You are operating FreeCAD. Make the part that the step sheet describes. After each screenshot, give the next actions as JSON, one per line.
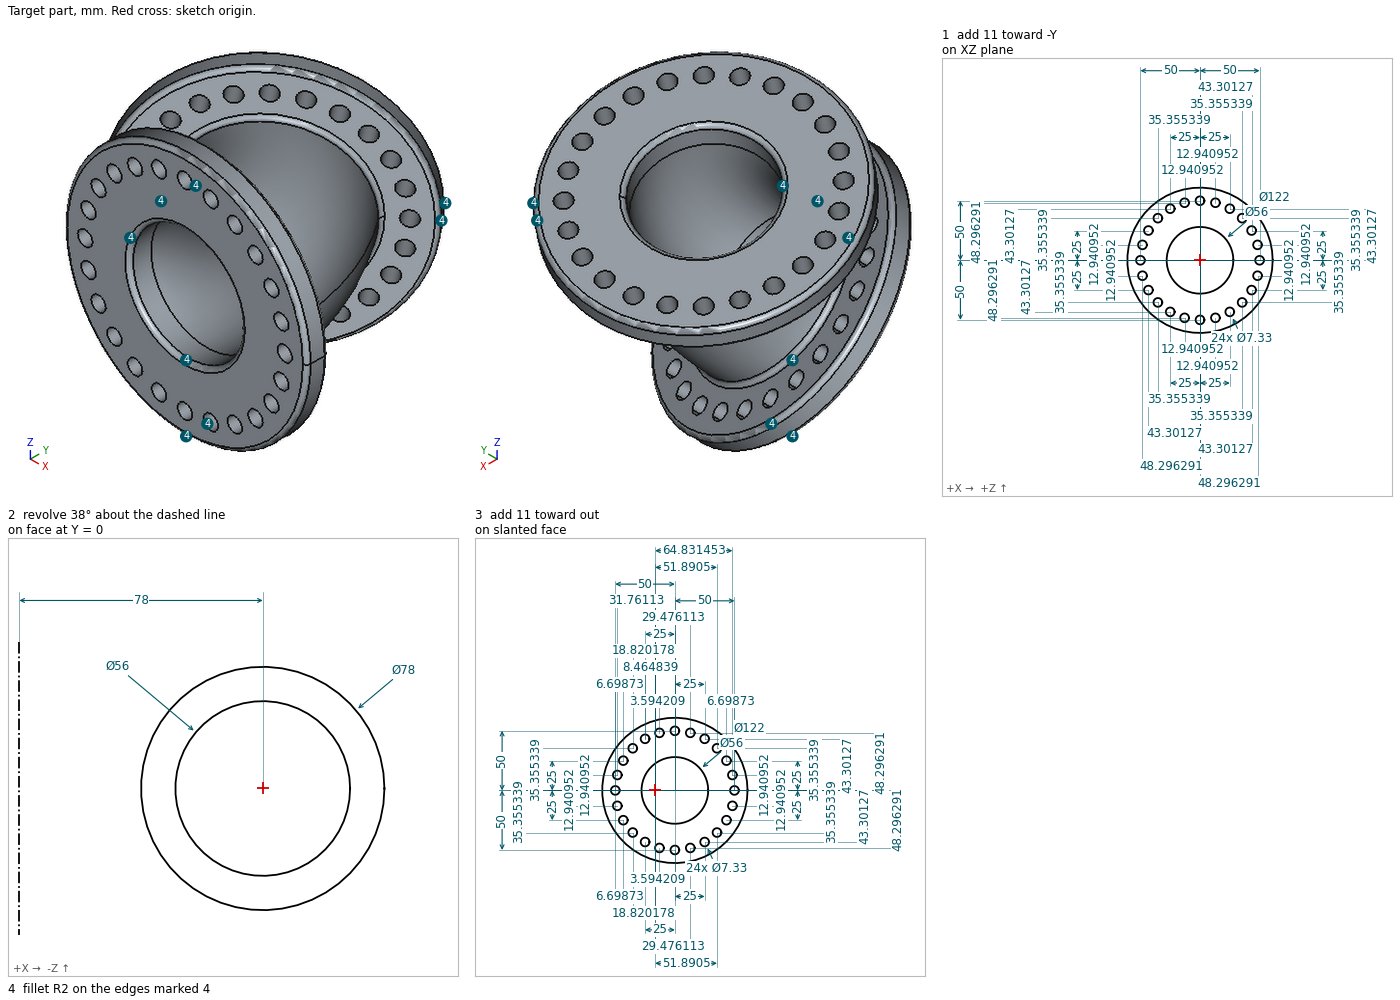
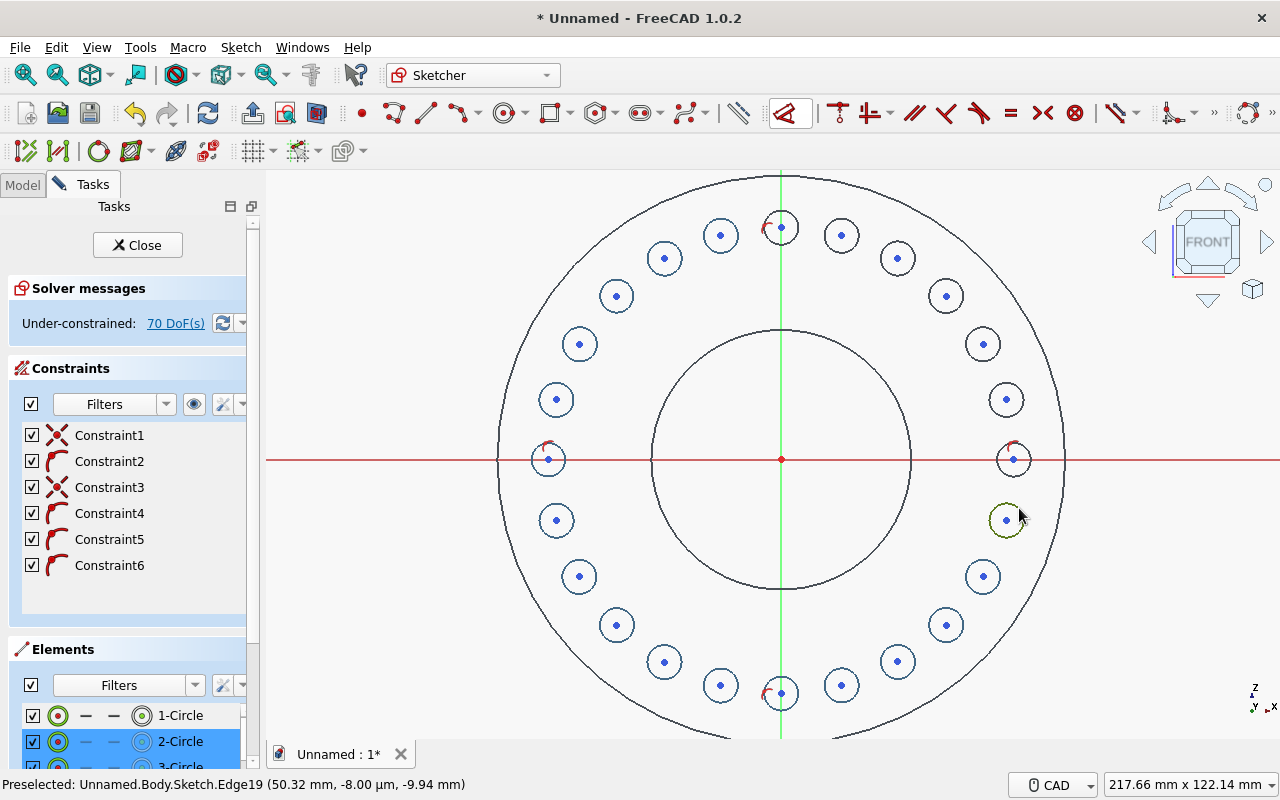
{"action": "left_click", "coordinate": [1026, 448]}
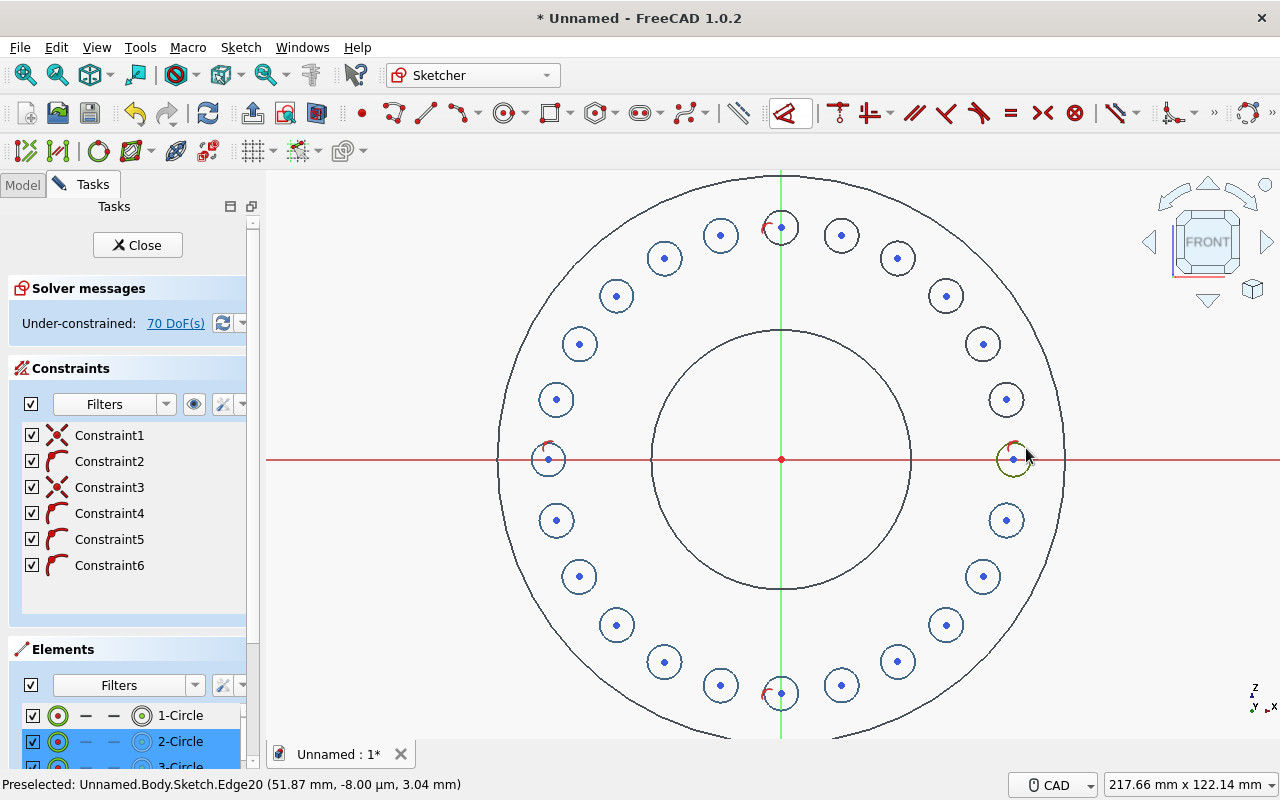
{"action": "left_click", "coordinate": [793, 216]}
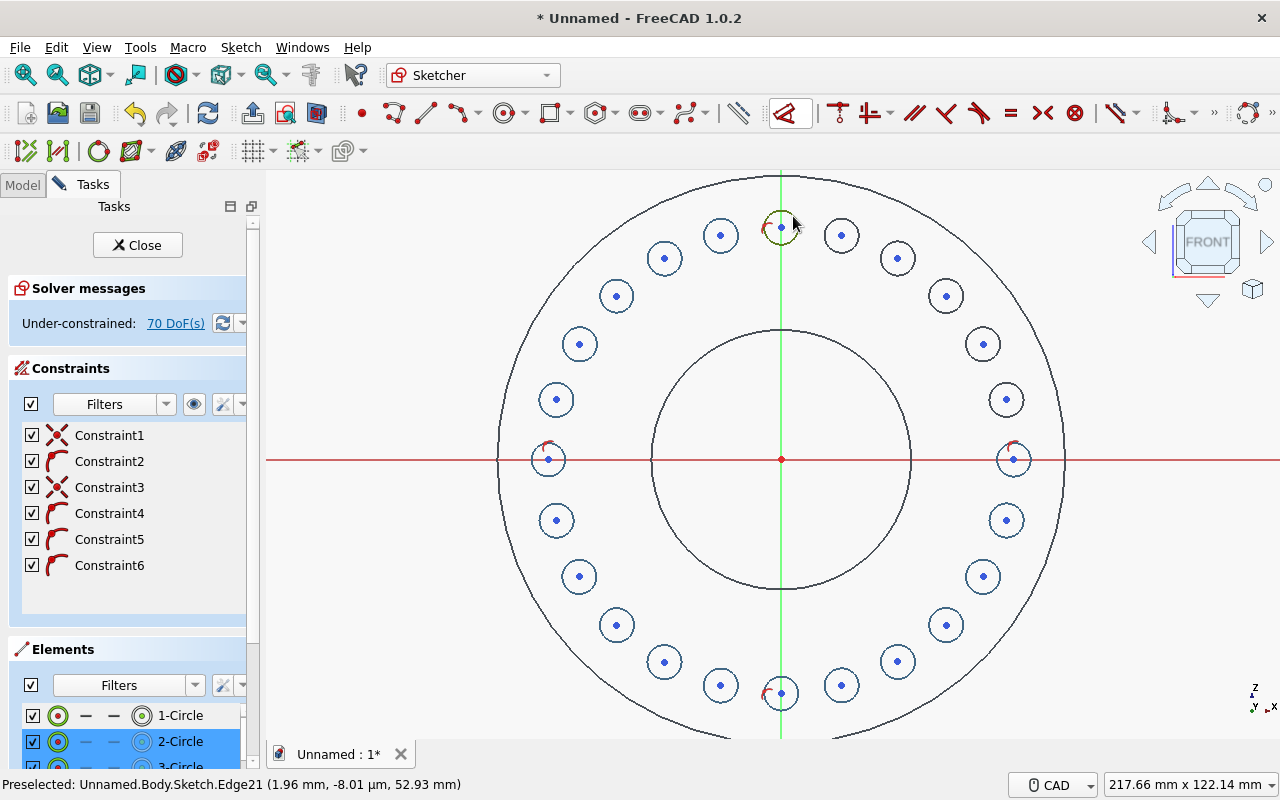
{"action": "left_click", "coordinate": [854, 224]}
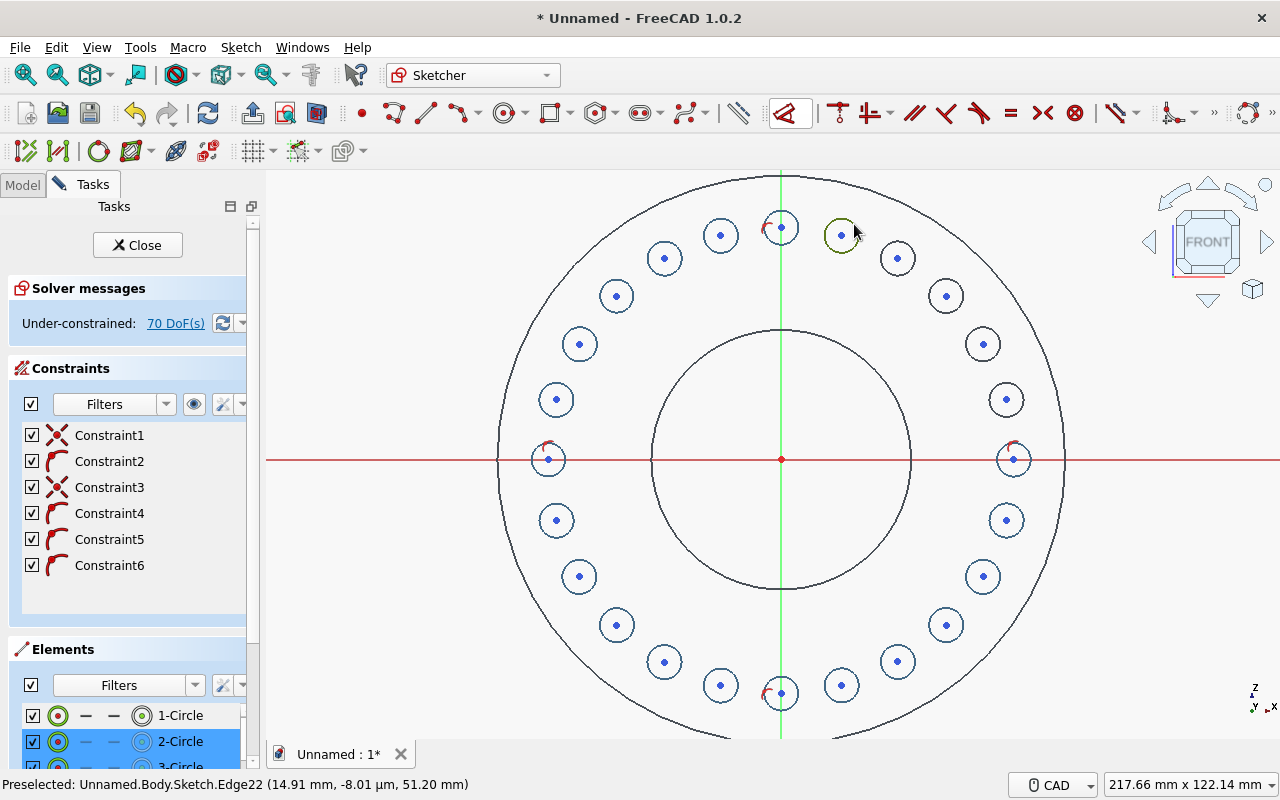
{"action": "left_click", "coordinate": [910, 246]}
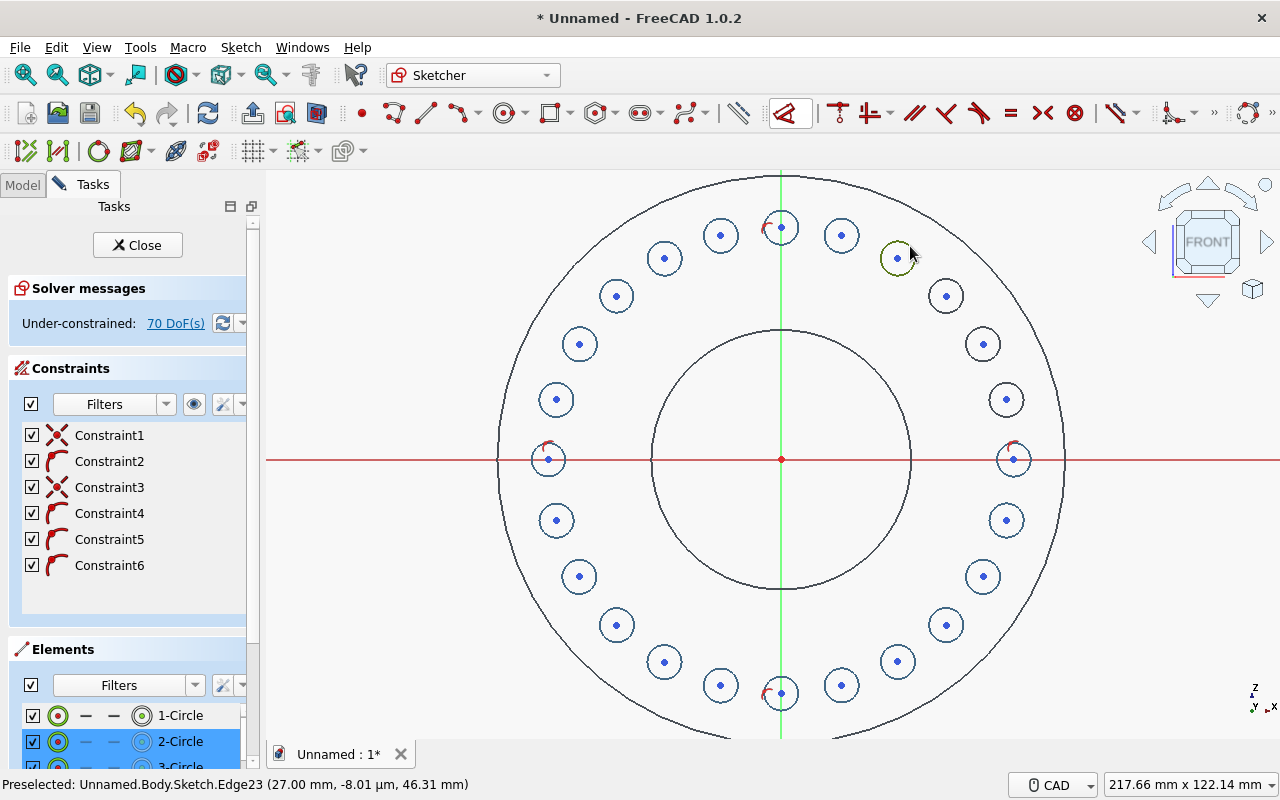
{"action": "left_click", "coordinate": [1019, 388]}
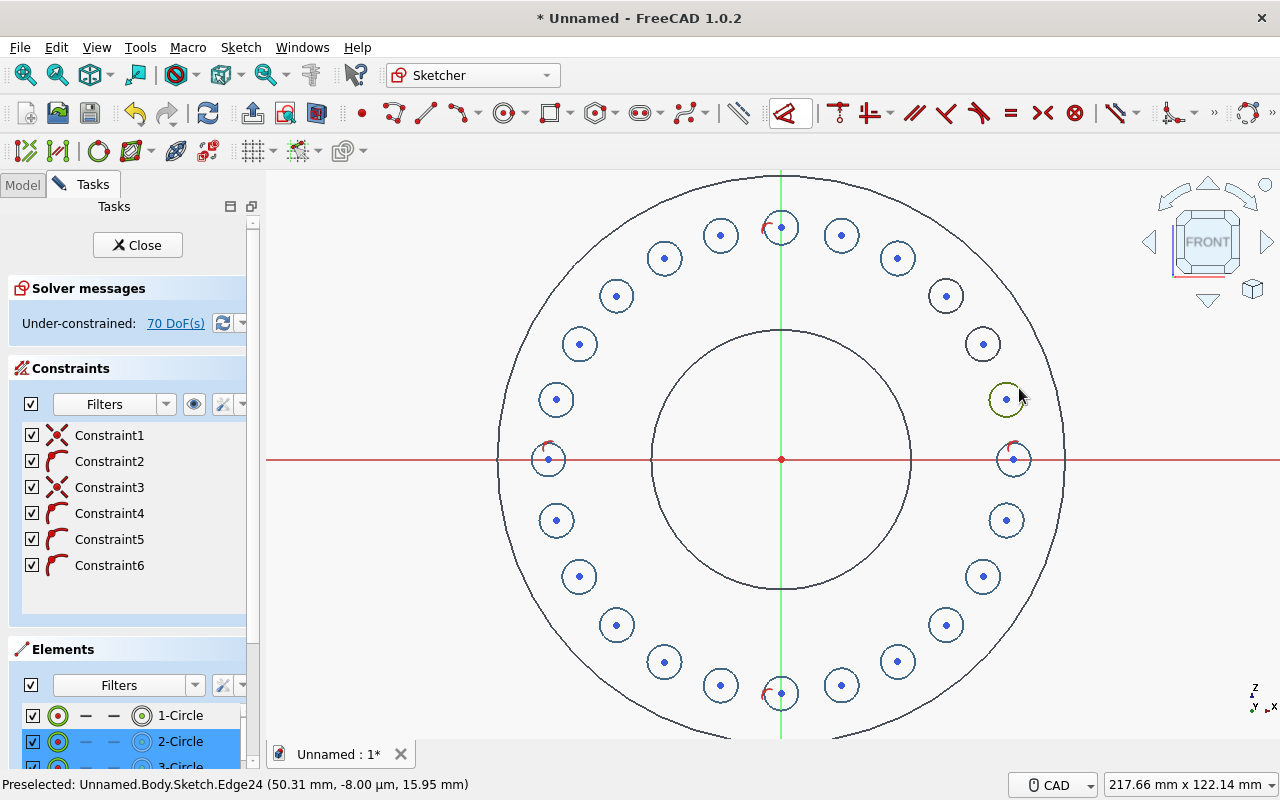
{"action": "left_click", "coordinate": [995, 332]}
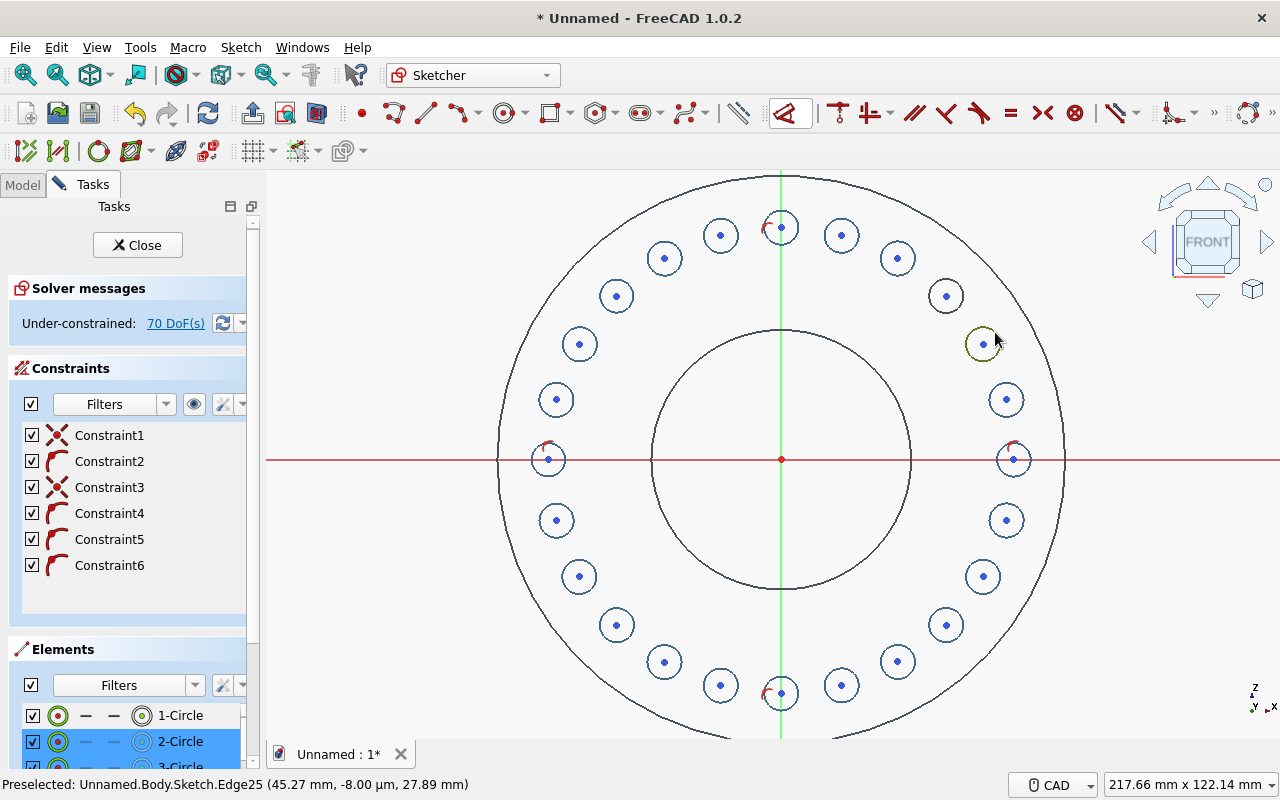
{"action": "left_click", "coordinate": [958, 284]}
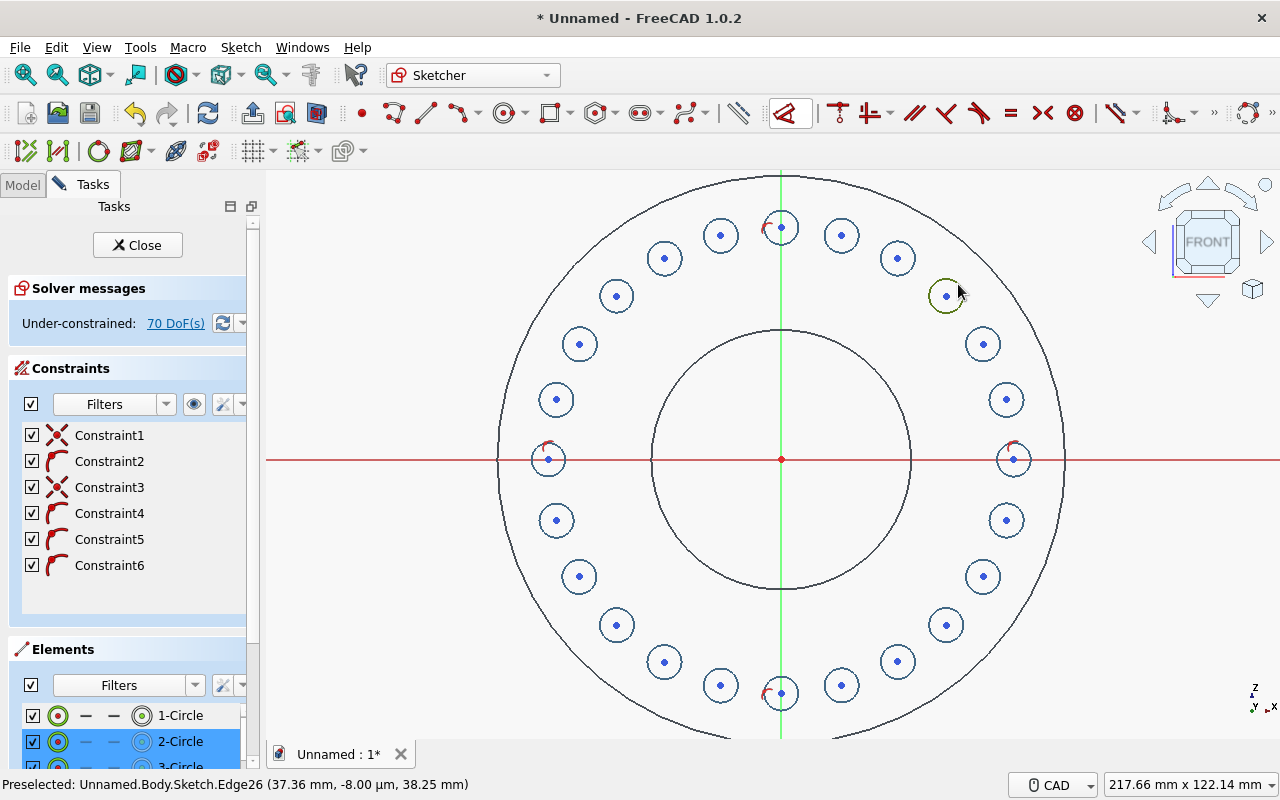
{"action": "left_click", "coordinate": [1012, 114]}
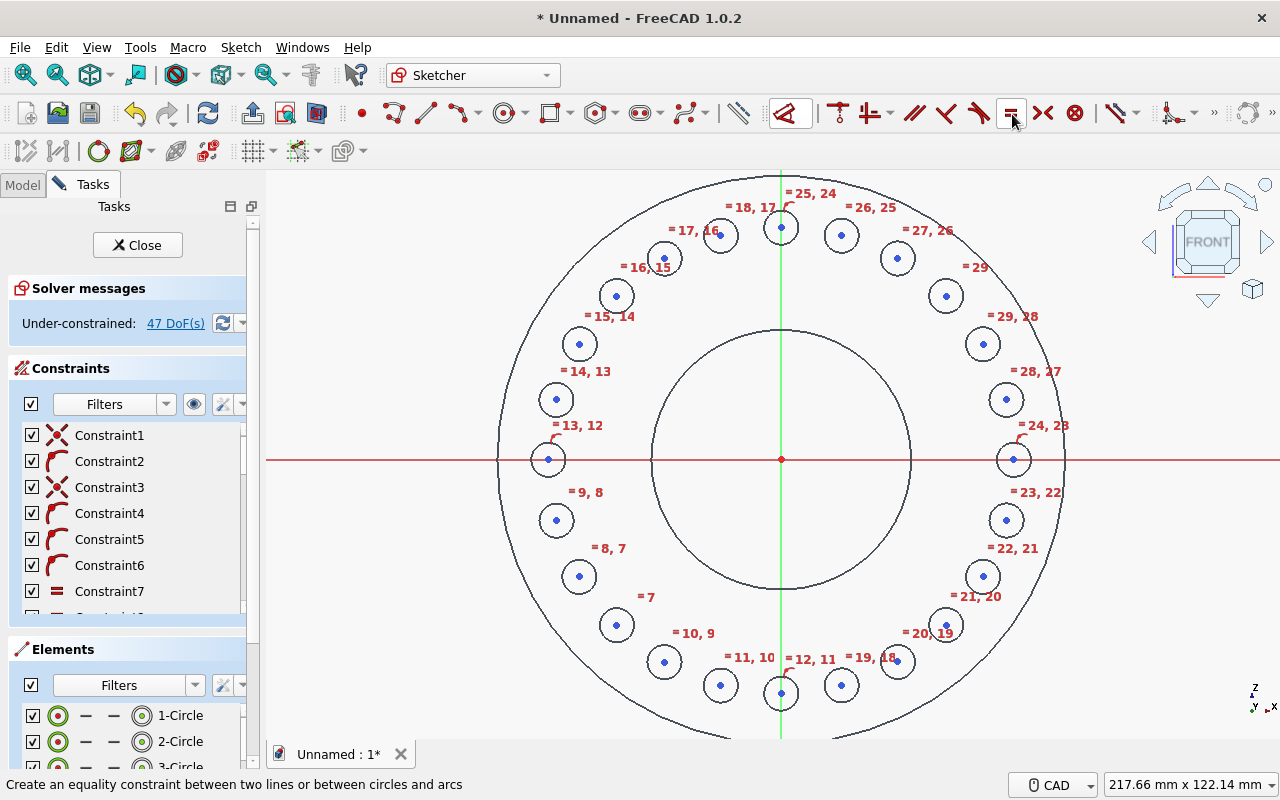
{"action": "left_click", "coordinate": [557, 521]}